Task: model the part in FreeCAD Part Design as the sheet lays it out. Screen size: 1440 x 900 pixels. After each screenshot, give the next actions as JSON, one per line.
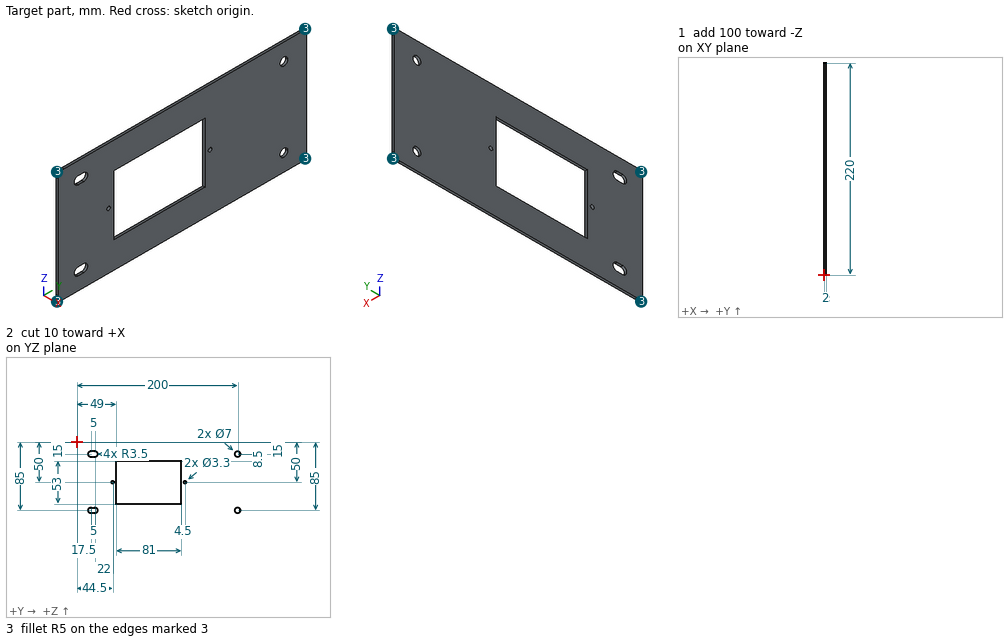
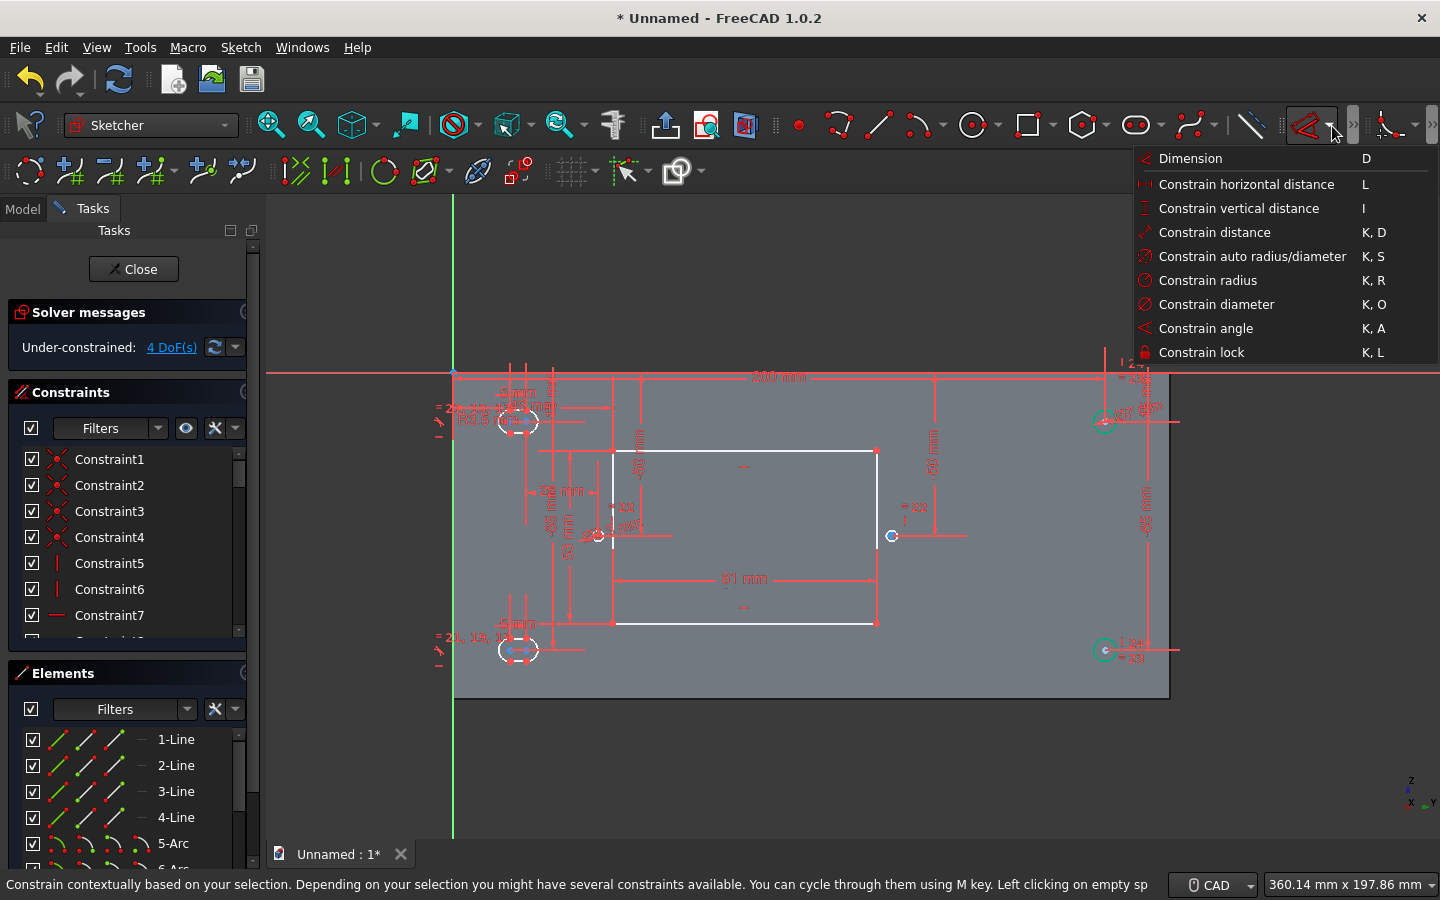
{"action": "left_click", "coordinate": [1286, 184]}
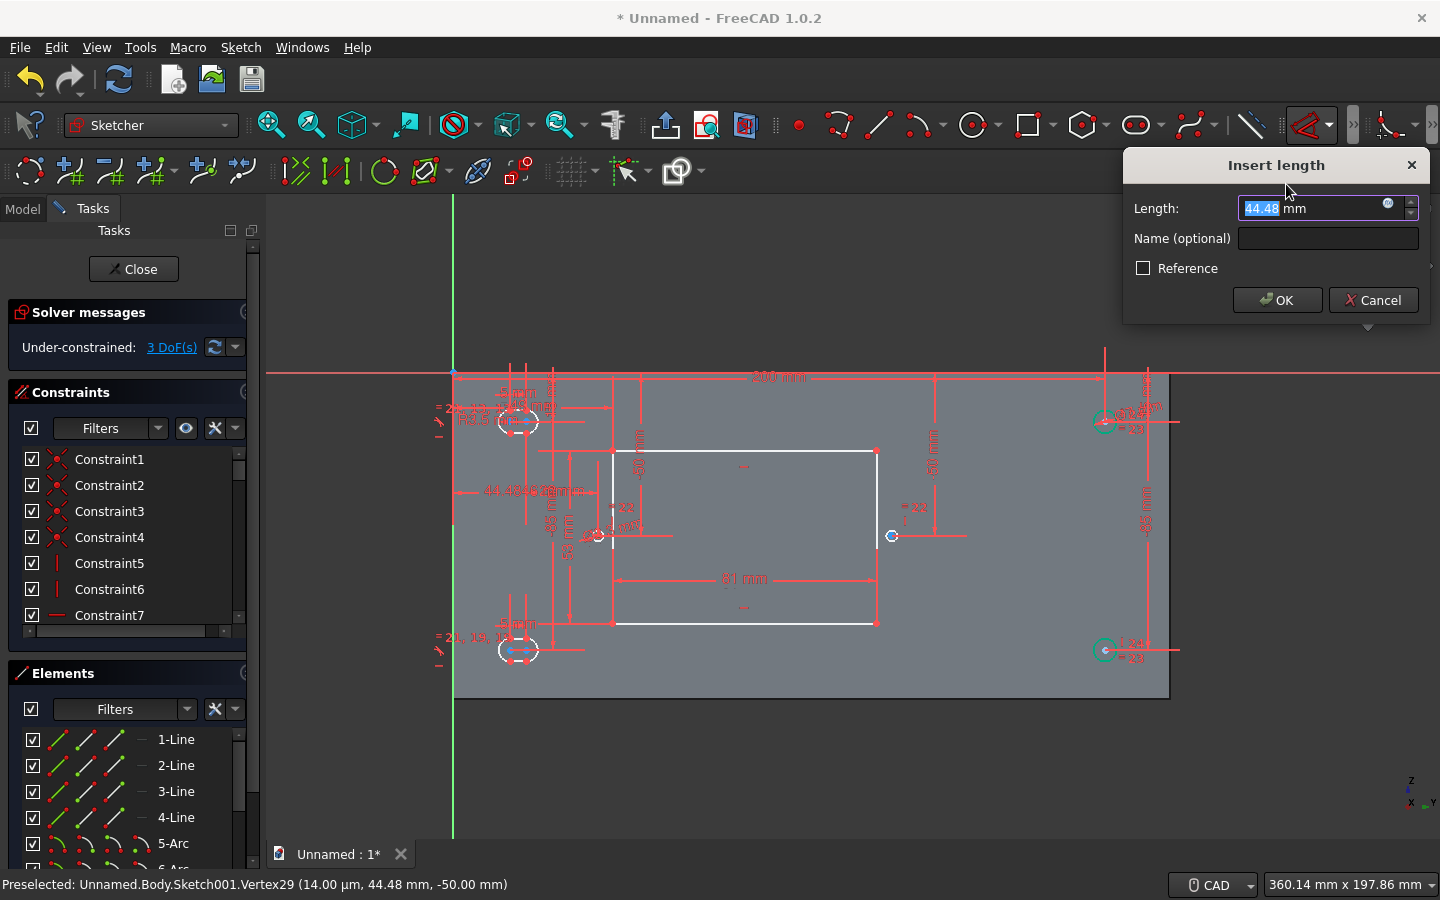
{"action": "type", "text": "44.5"}
{"action": "key", "text": "Return"}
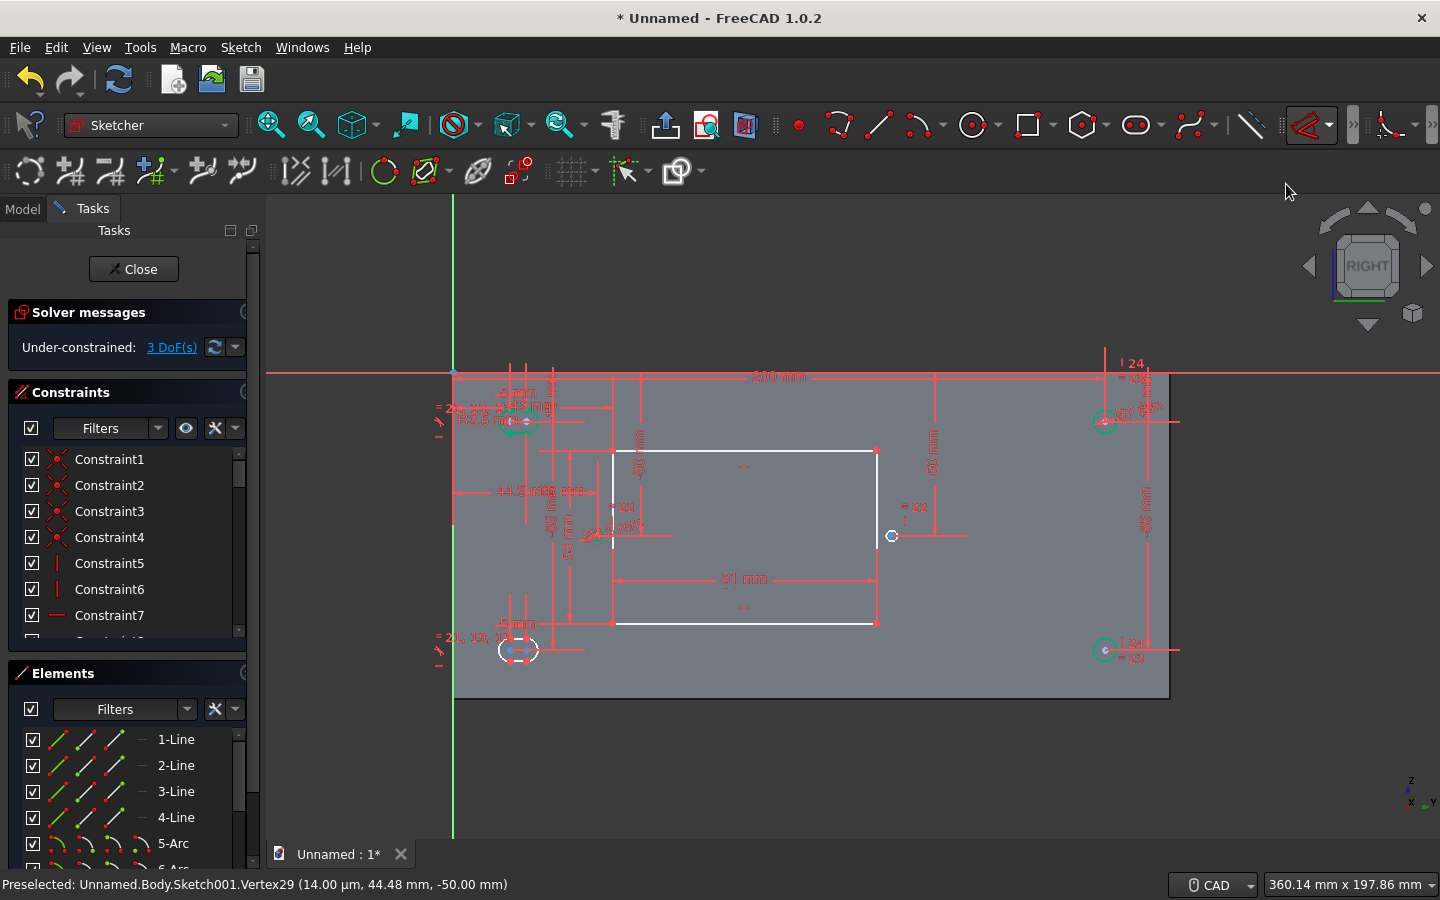
{"action": "scroll", "coordinate": [877, 624], "scroll_direction": "up", "scroll_amount": 5}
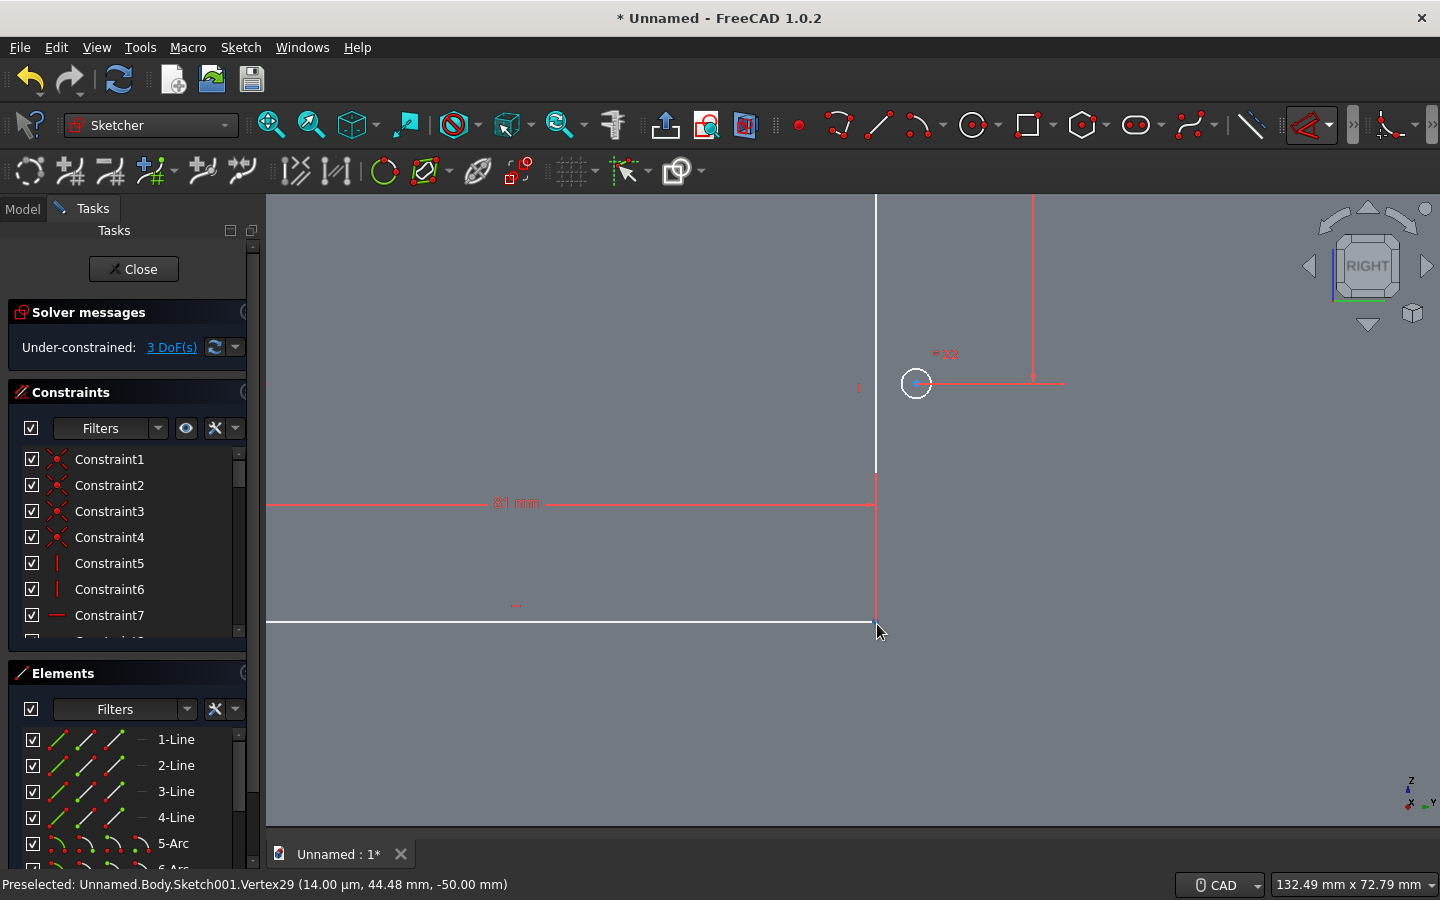
{"action": "left_click", "coordinate": [876, 622]}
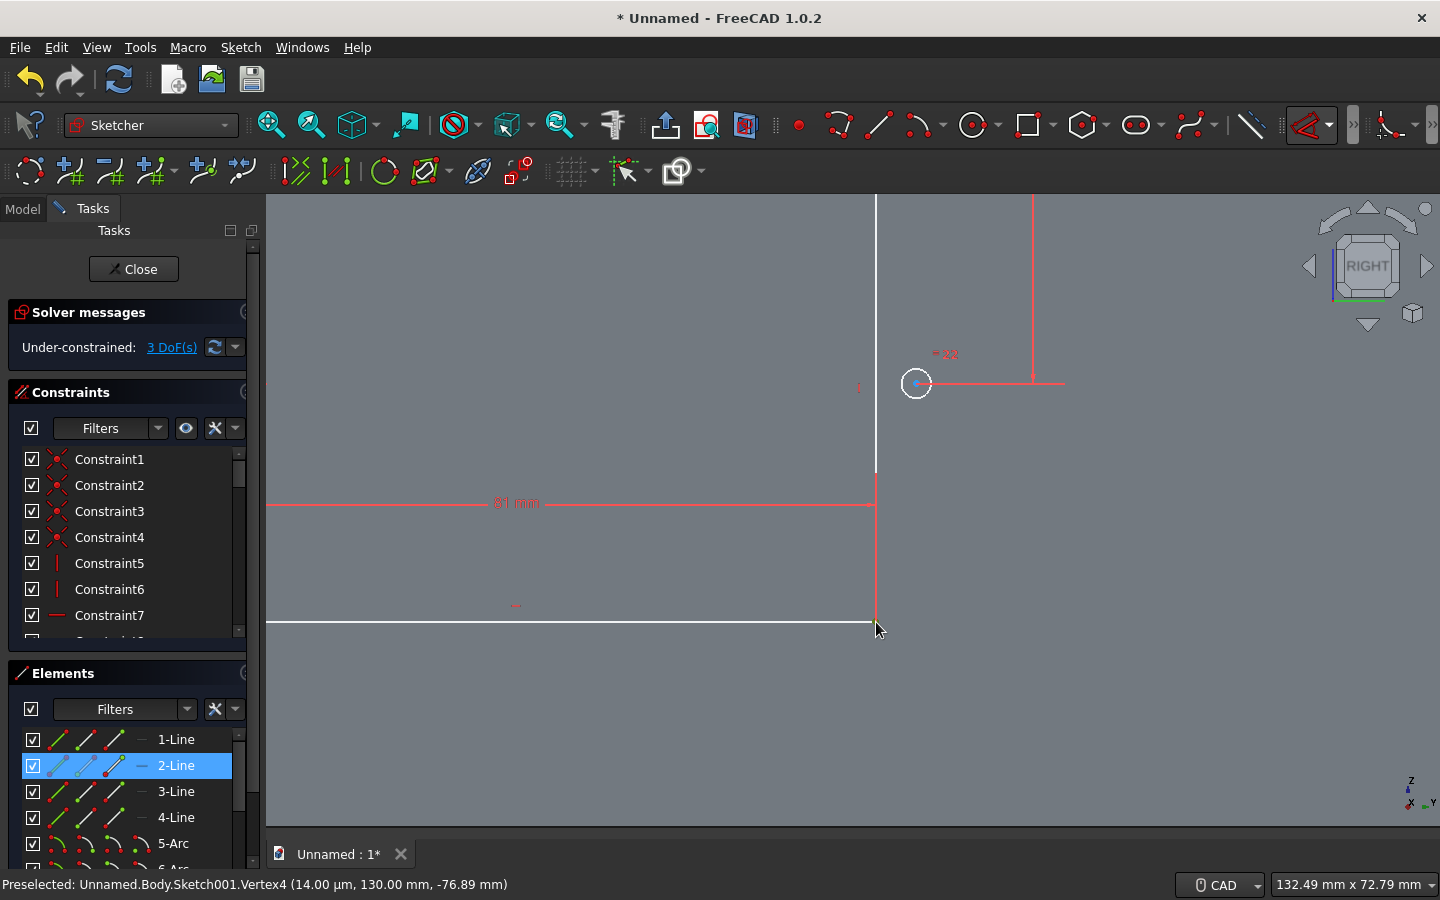
{"action": "left_click", "coordinate": [916, 384]}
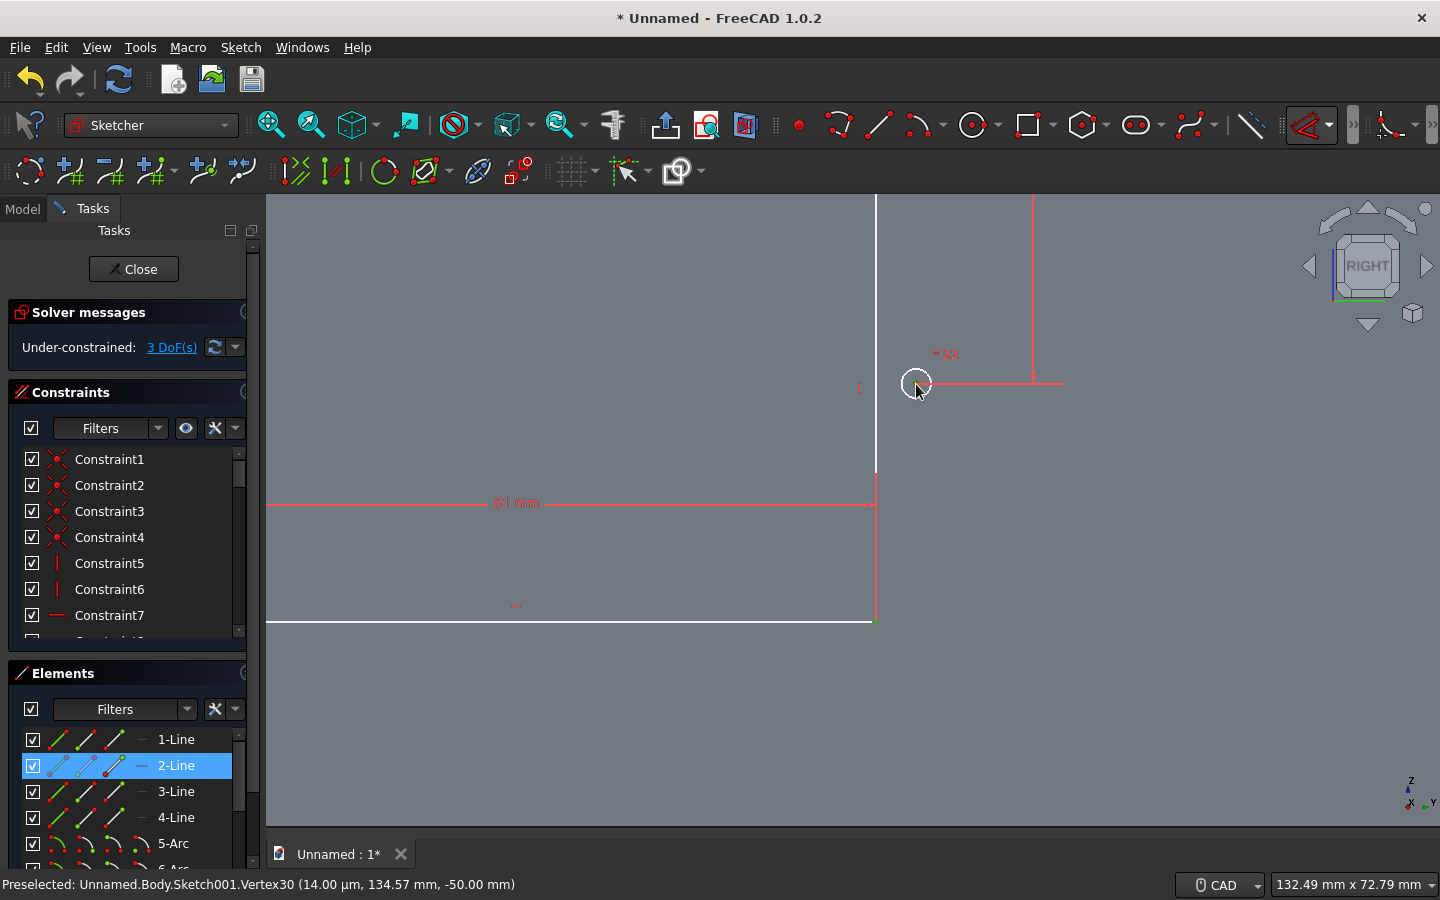
{"action": "left_click", "coordinate": [1332, 126]}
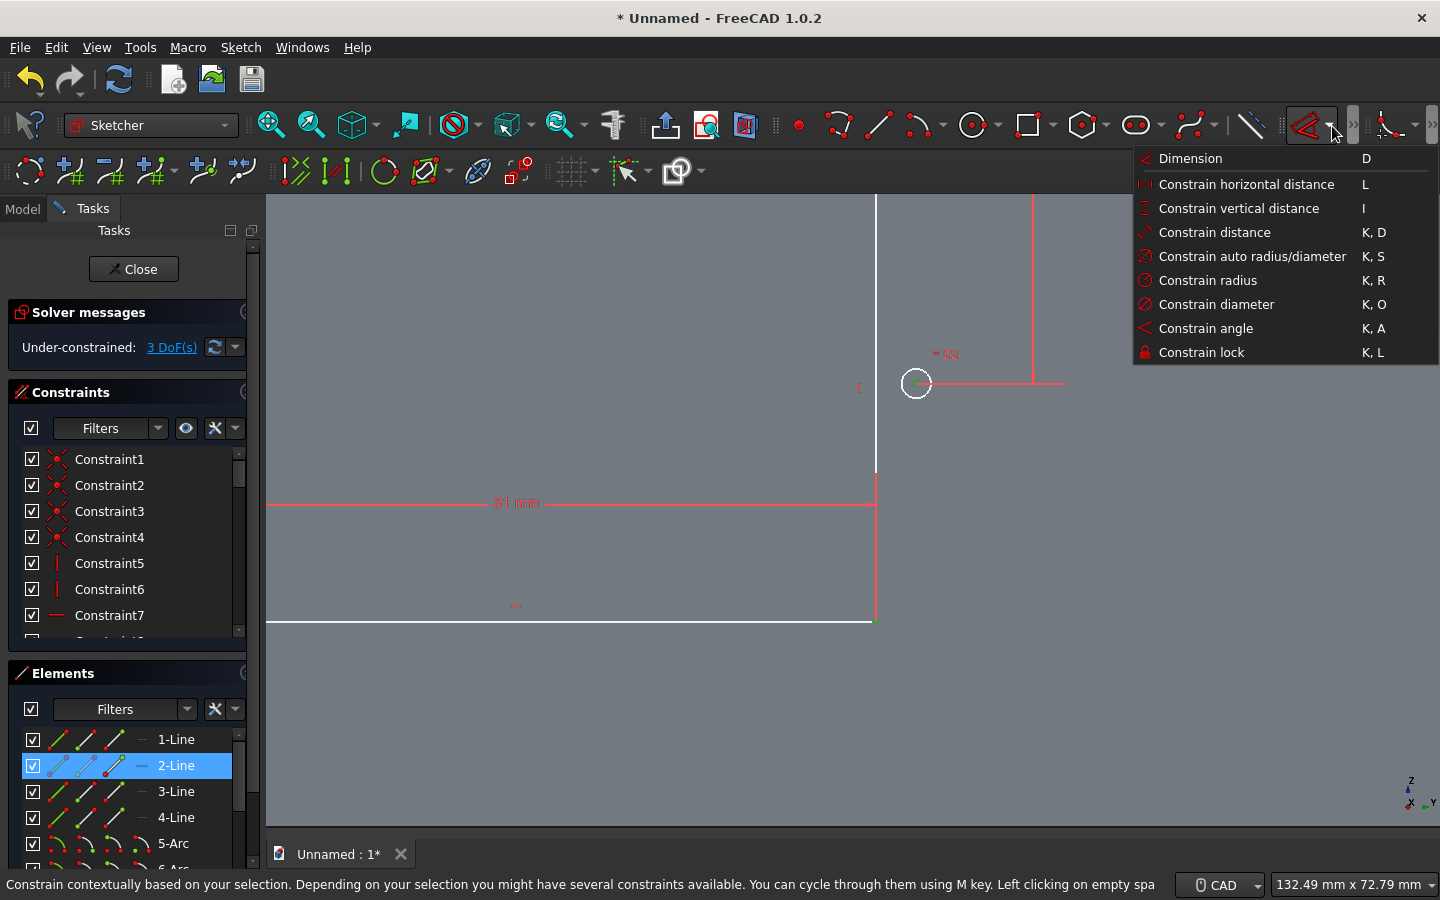
{"action": "left_click", "coordinate": [1286, 184]}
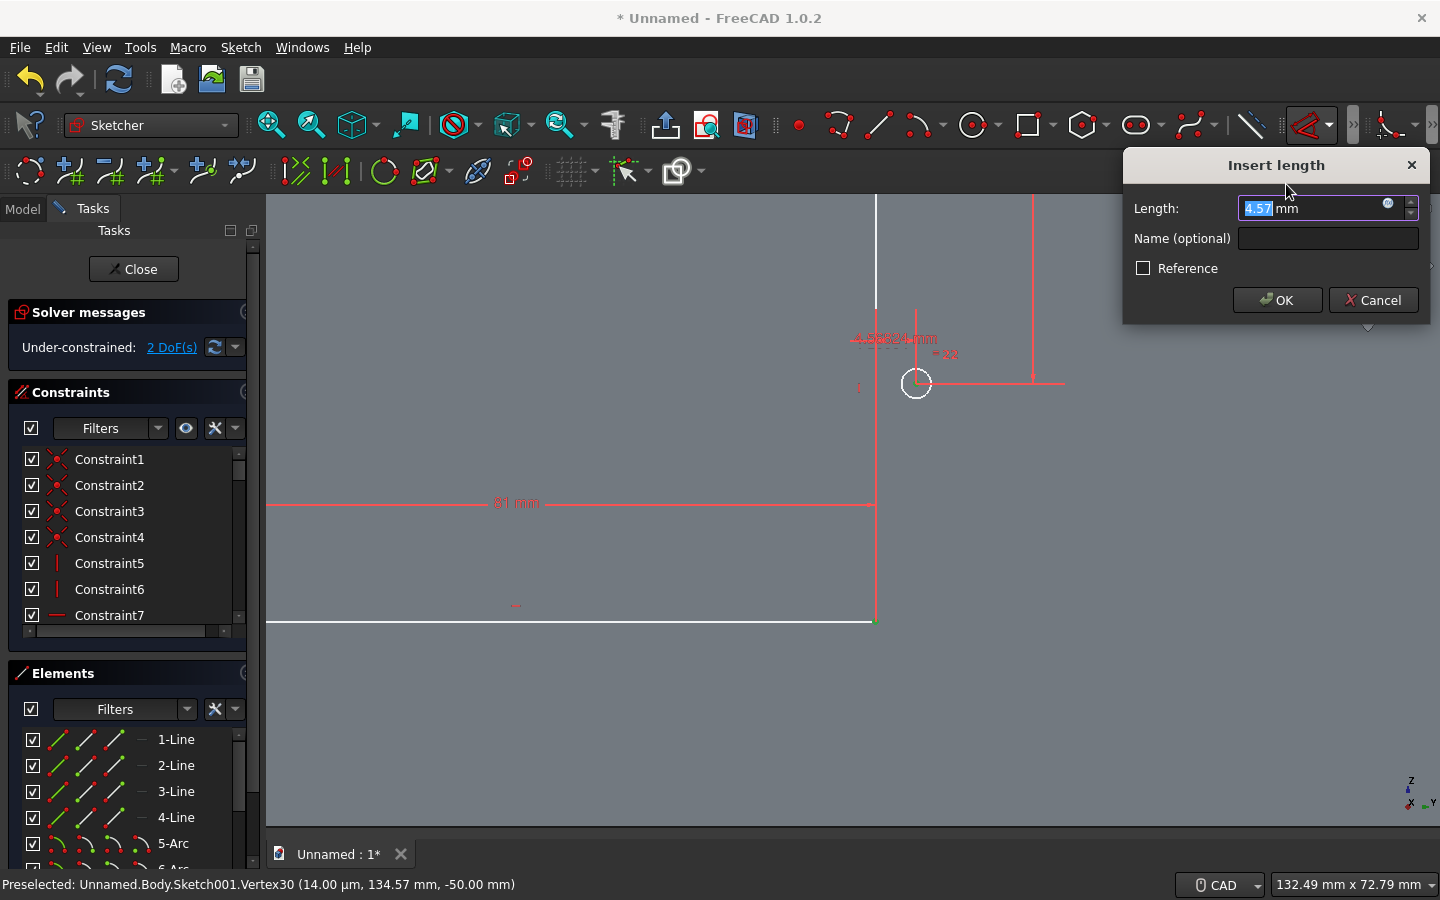
{"action": "type", "text": "4.5"}
{"action": "key", "text": "Return"}